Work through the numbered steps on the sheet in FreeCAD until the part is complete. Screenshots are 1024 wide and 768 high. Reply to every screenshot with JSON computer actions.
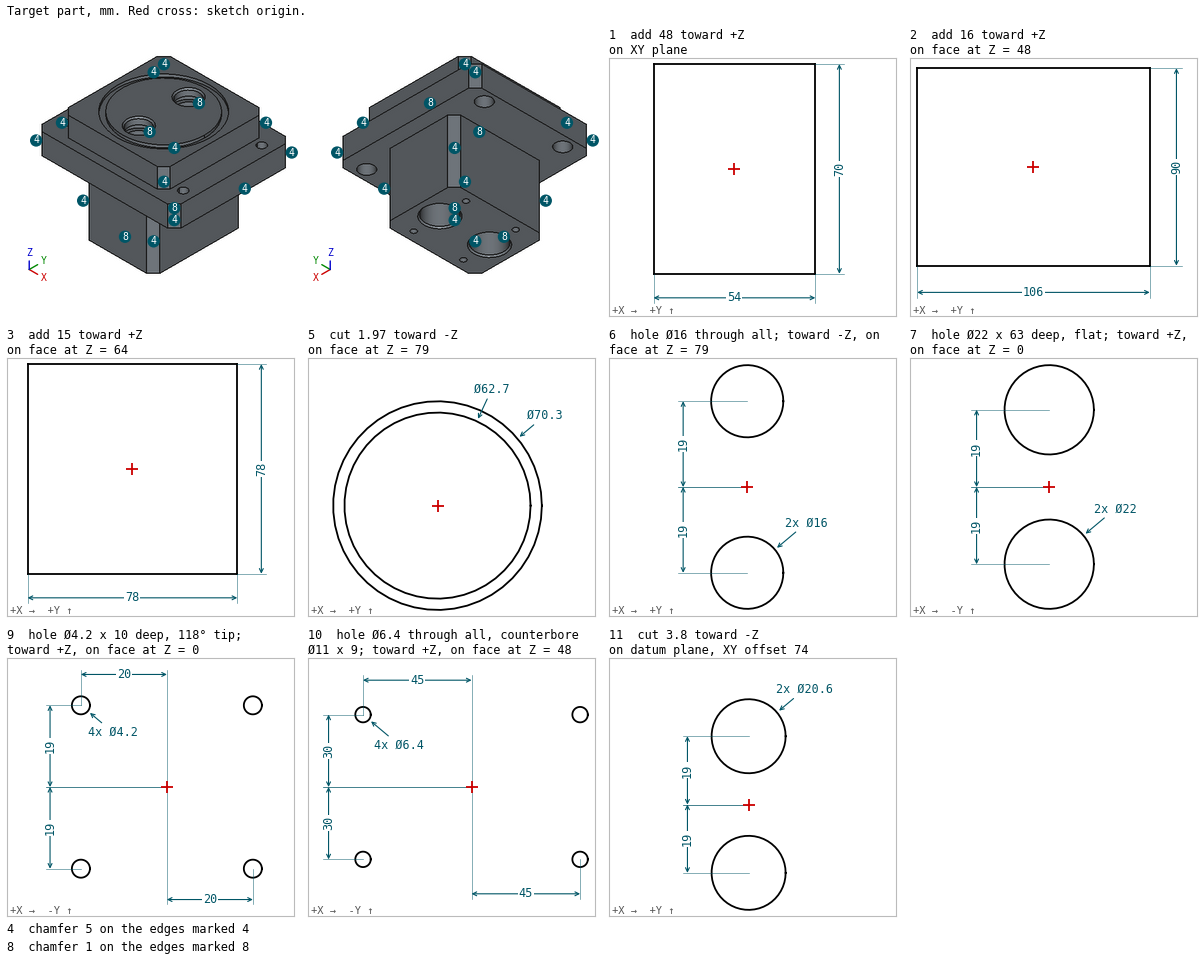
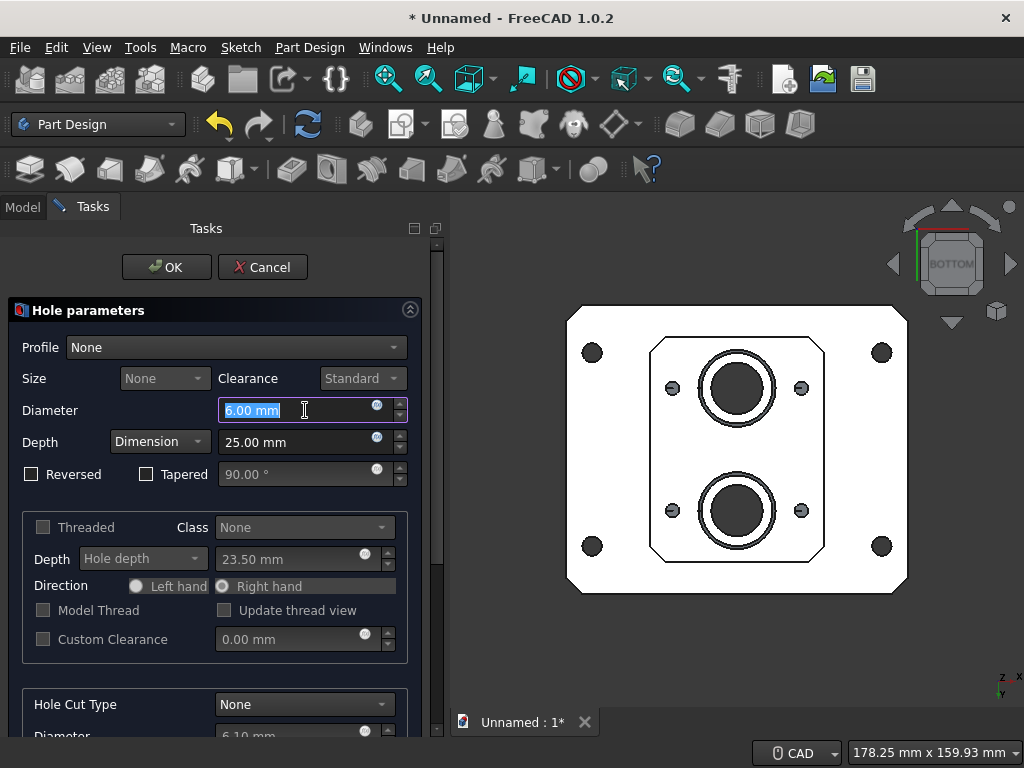
{"action": "type", "text": "6.4"}
{"action": "key", "text": "Tab"}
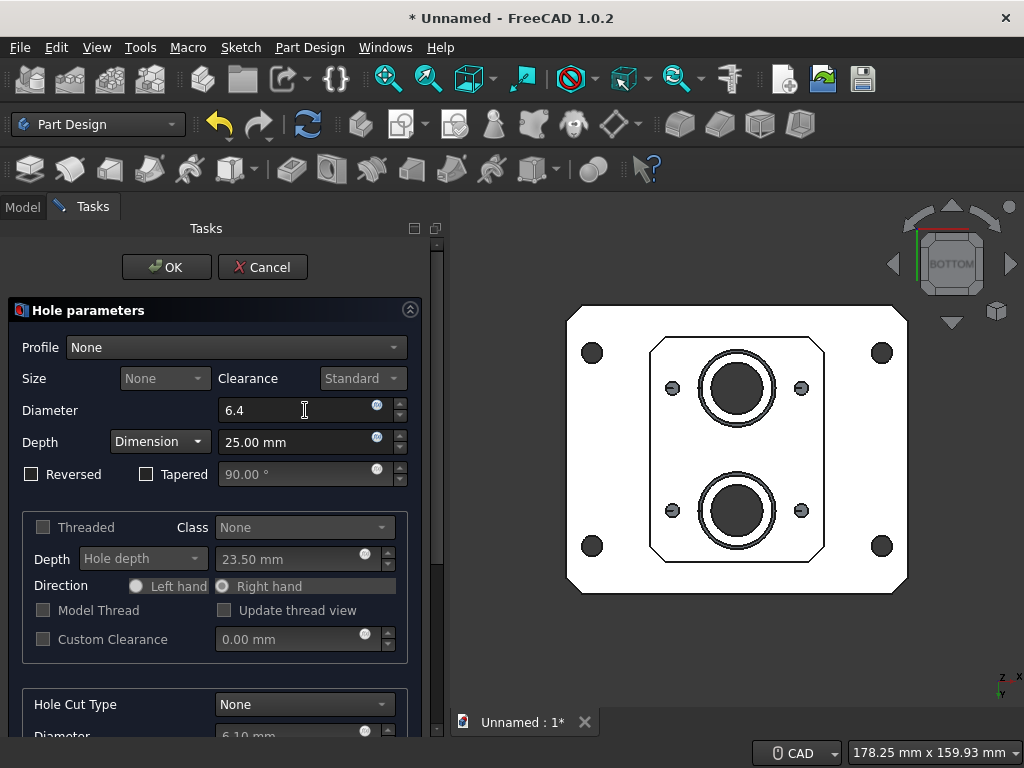
{"action": "left_click", "coordinate": [161, 442]}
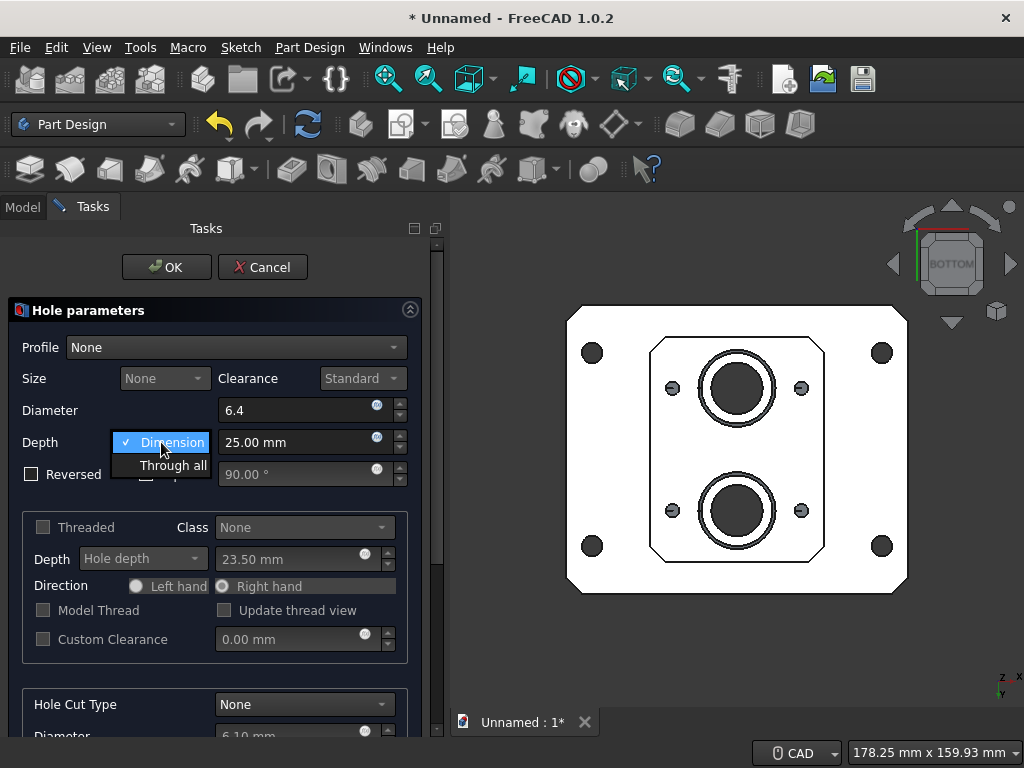
{"action": "left_click", "coordinate": [160, 466]}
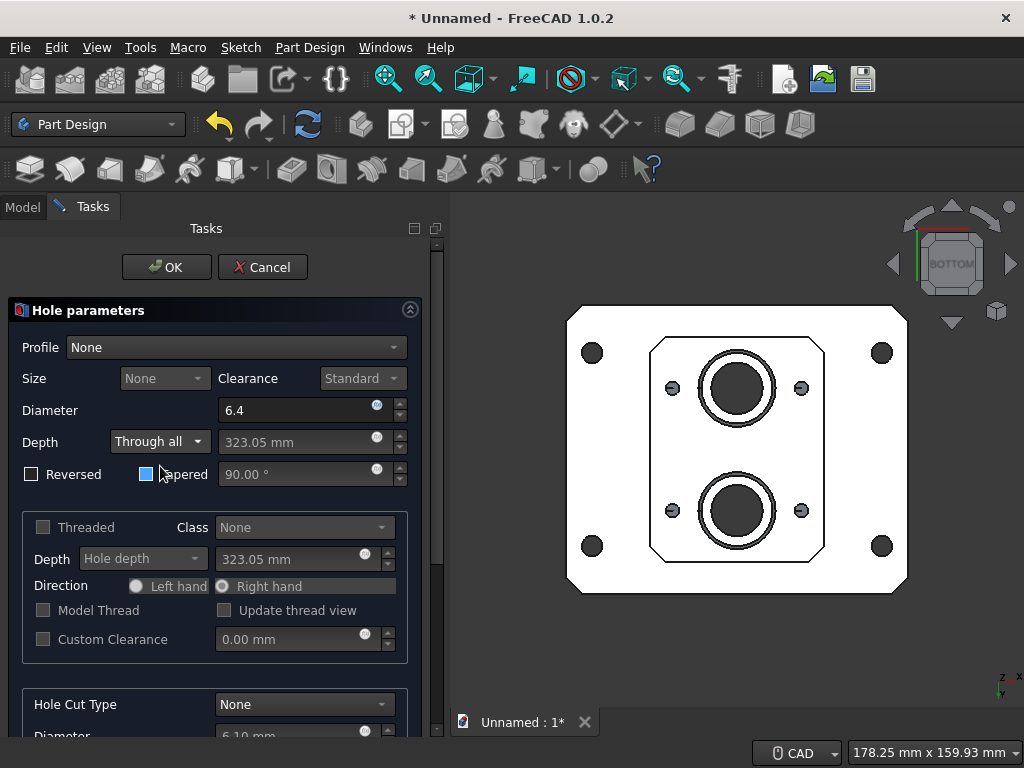
{"action": "left_click", "coordinate": [306, 704]}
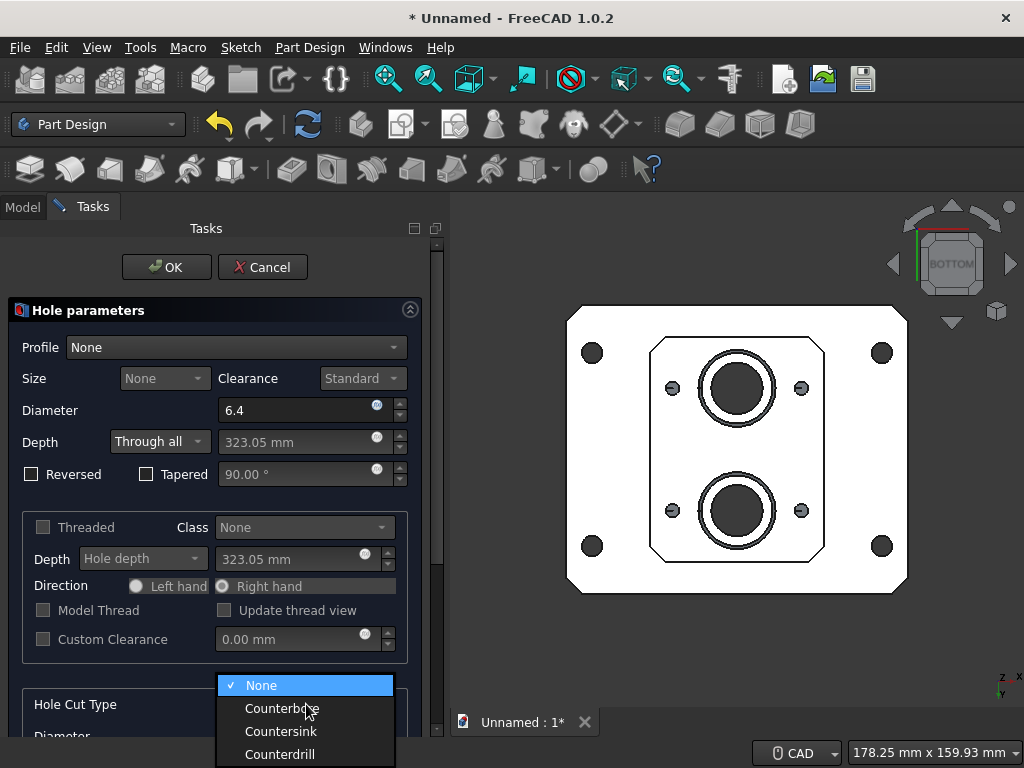
{"action": "left_click", "coordinate": [304, 708]}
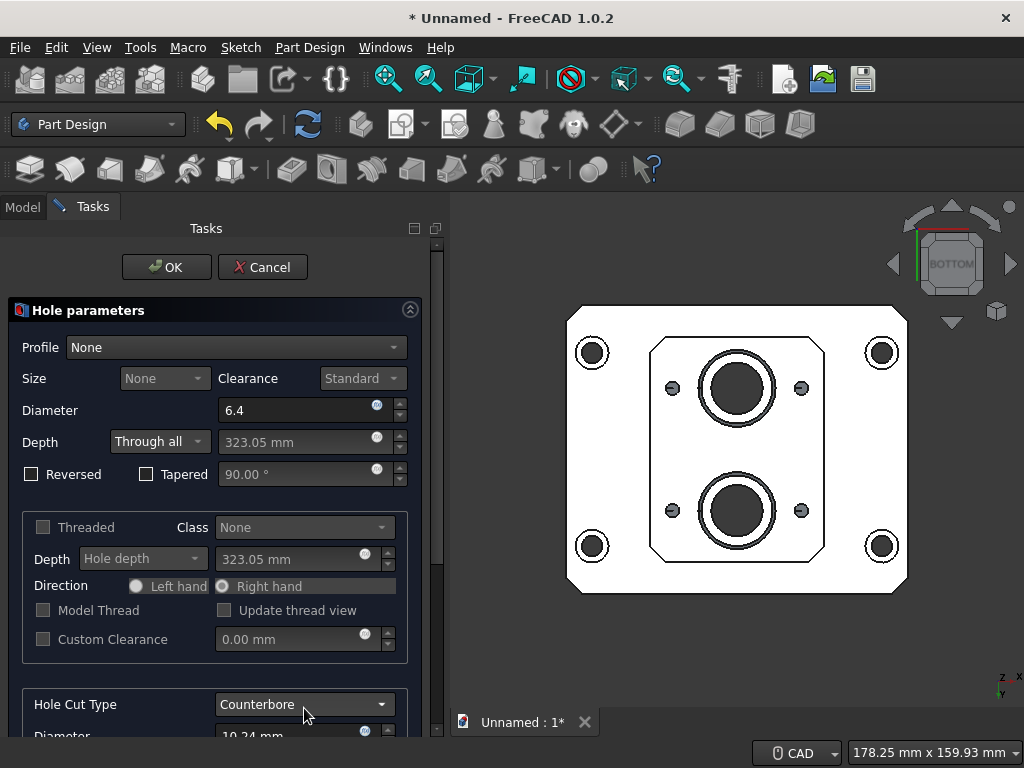
{"action": "scroll", "coordinate": [437, 487], "scroll_direction": "down", "scroll_amount": 2}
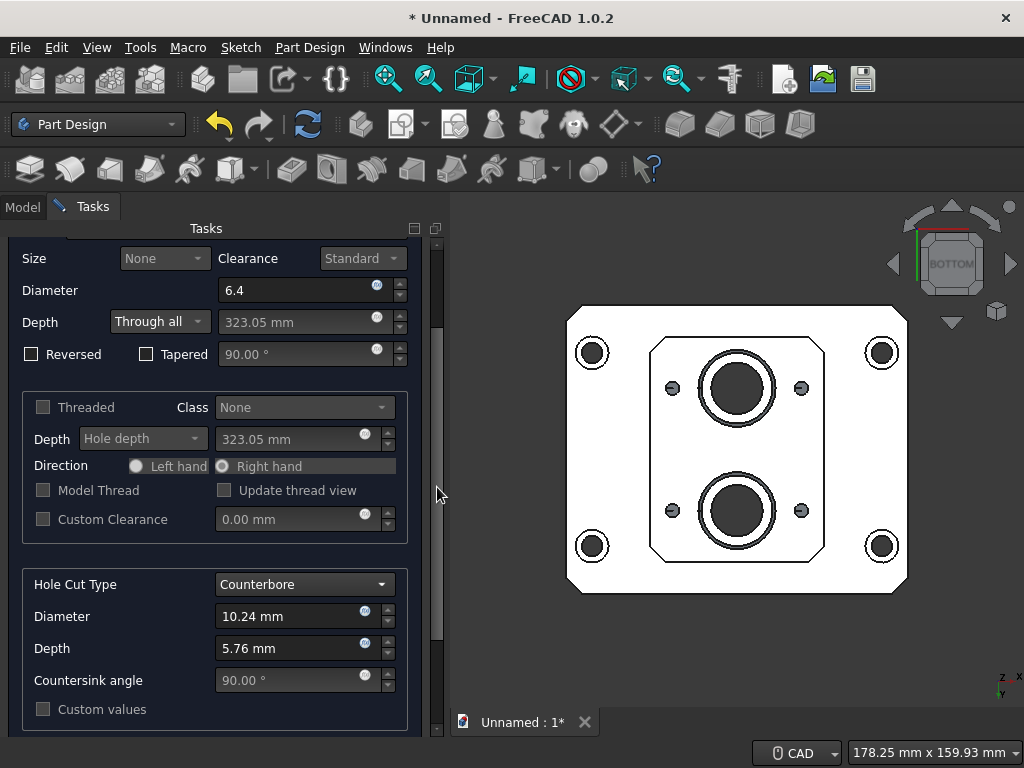
{"action": "triple_click", "coordinate": [298, 616]}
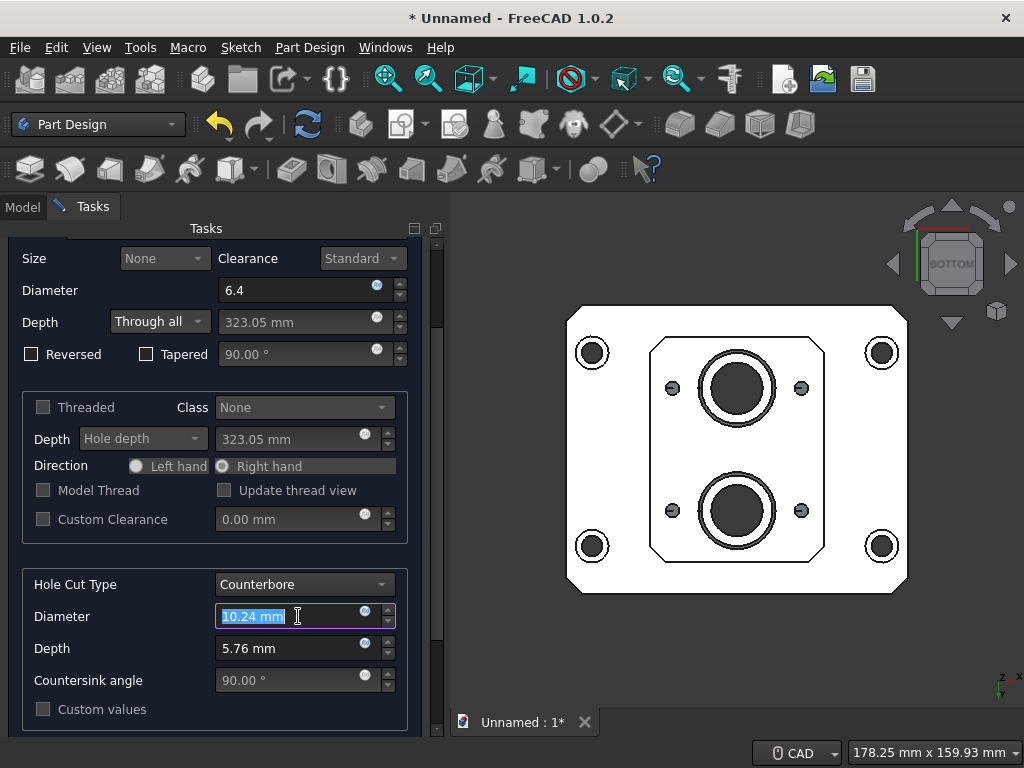
{"action": "type", "text": "11"}
{"action": "key", "text": "Tab"}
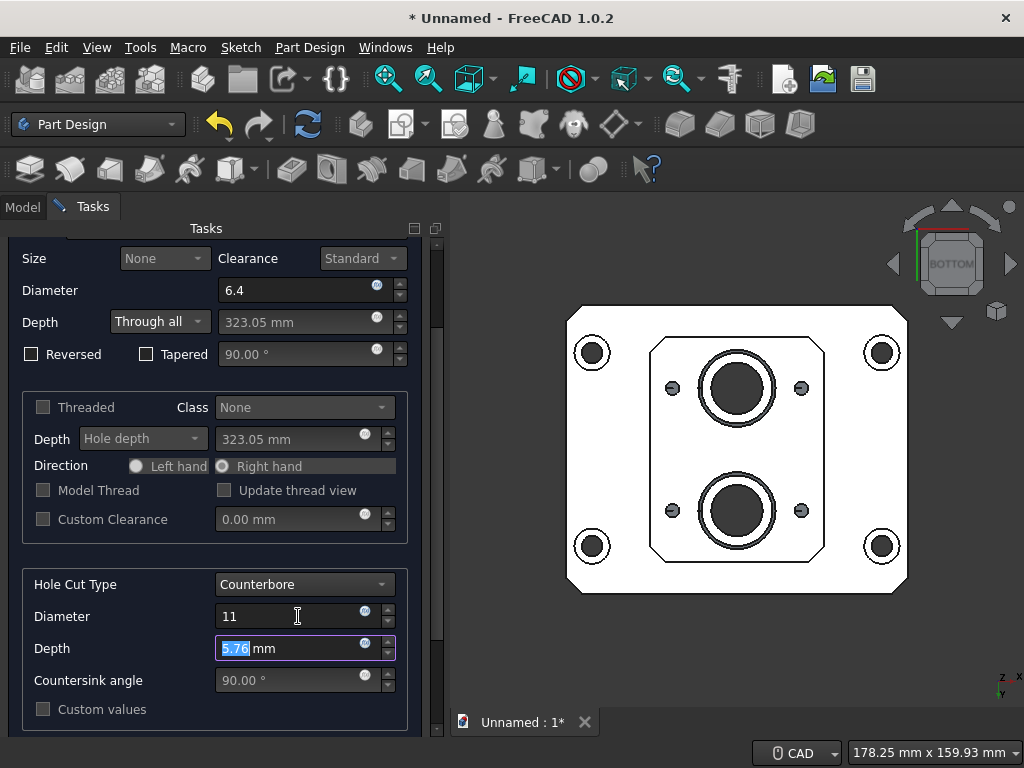
{"action": "type", "text": "9"}
{"action": "key", "text": "Tab"}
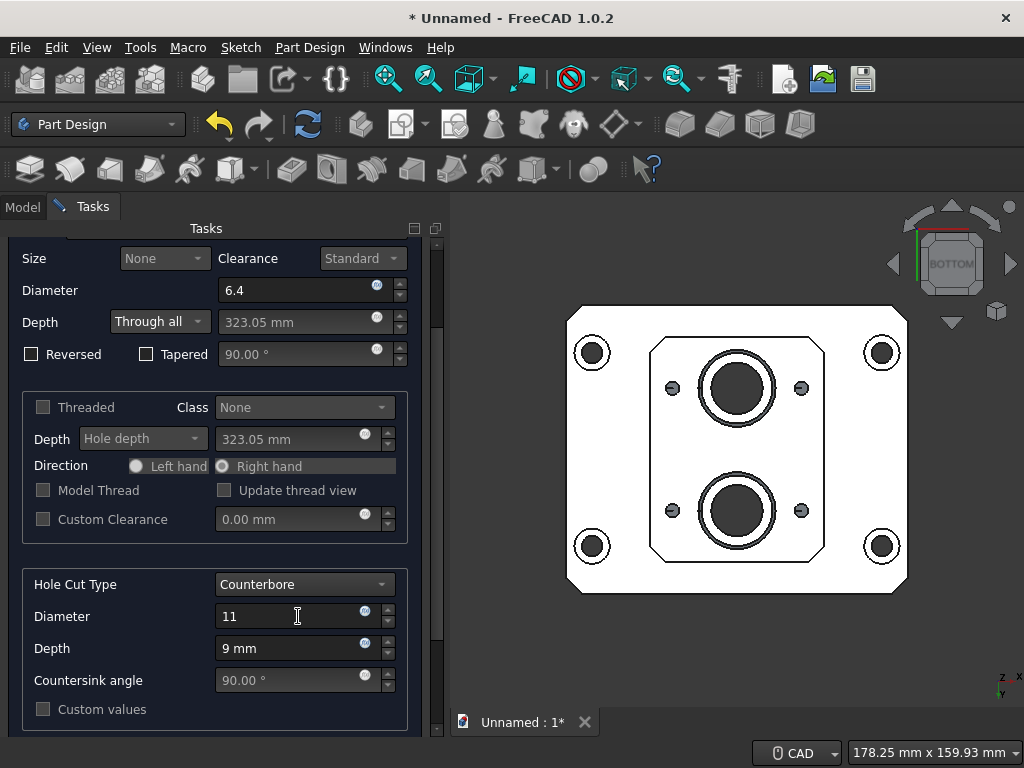
{"action": "scroll", "coordinate": [437, 487], "scroll_direction": "up", "scroll_amount": 3}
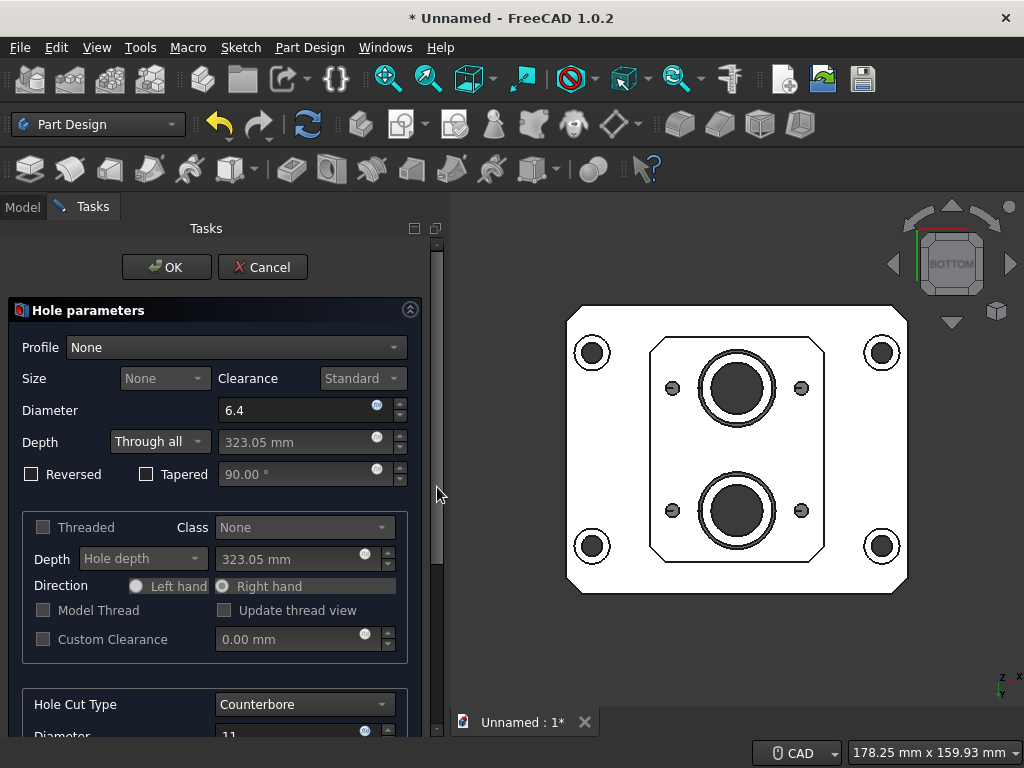
{"action": "left_click", "coordinate": [167, 267]}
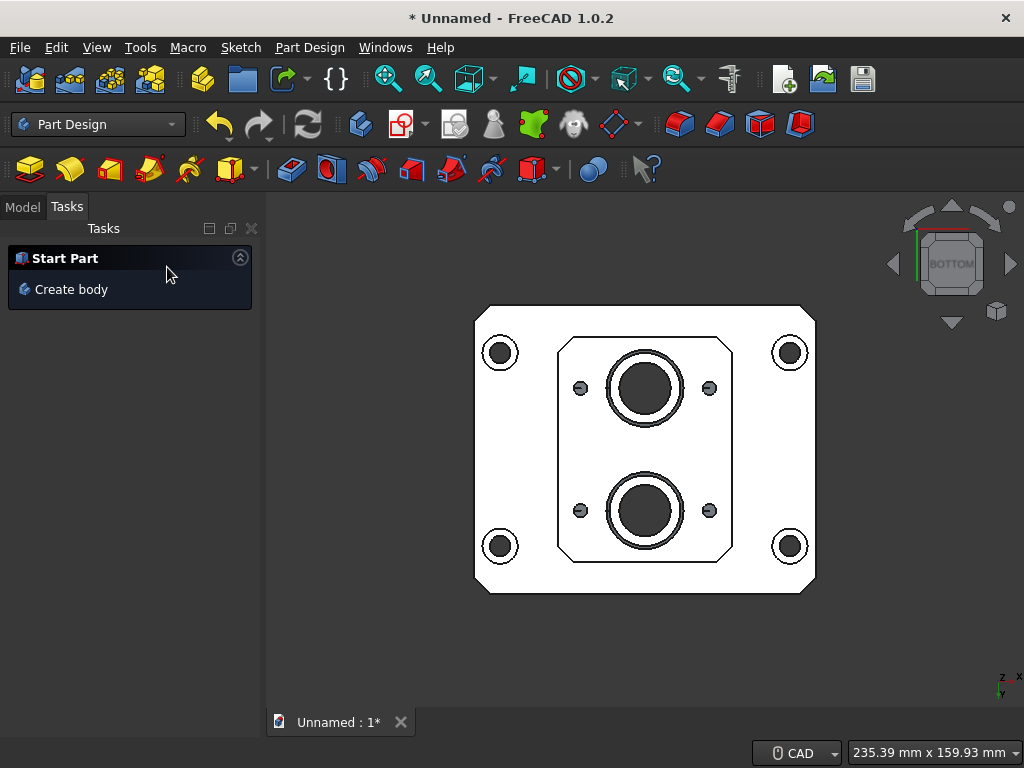
{"action": "left_click", "coordinate": [23, 206]}